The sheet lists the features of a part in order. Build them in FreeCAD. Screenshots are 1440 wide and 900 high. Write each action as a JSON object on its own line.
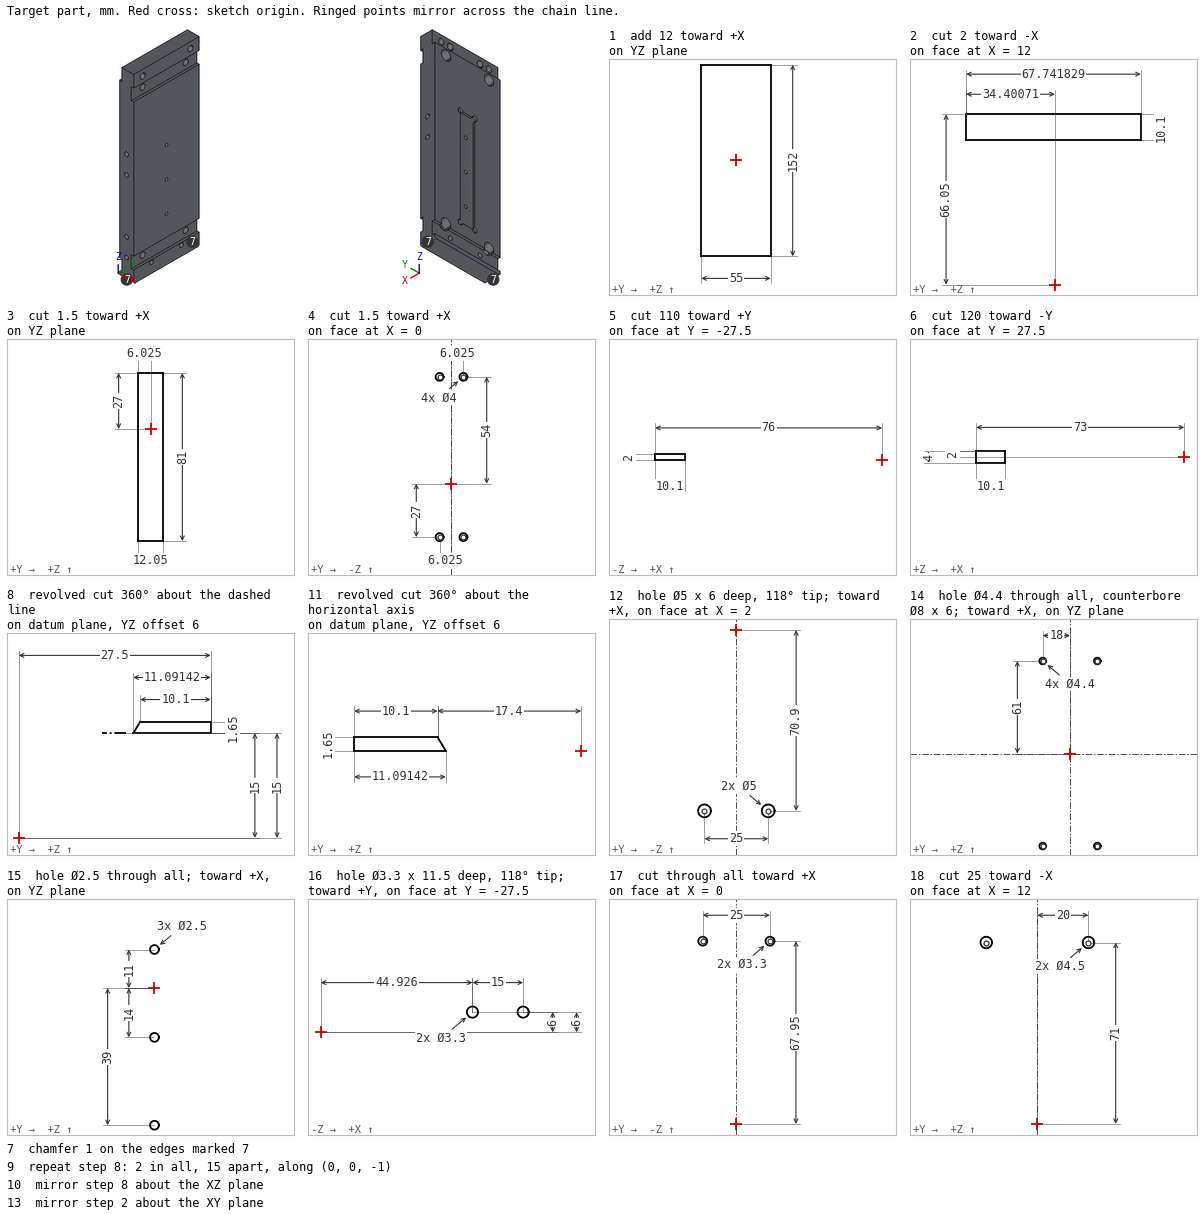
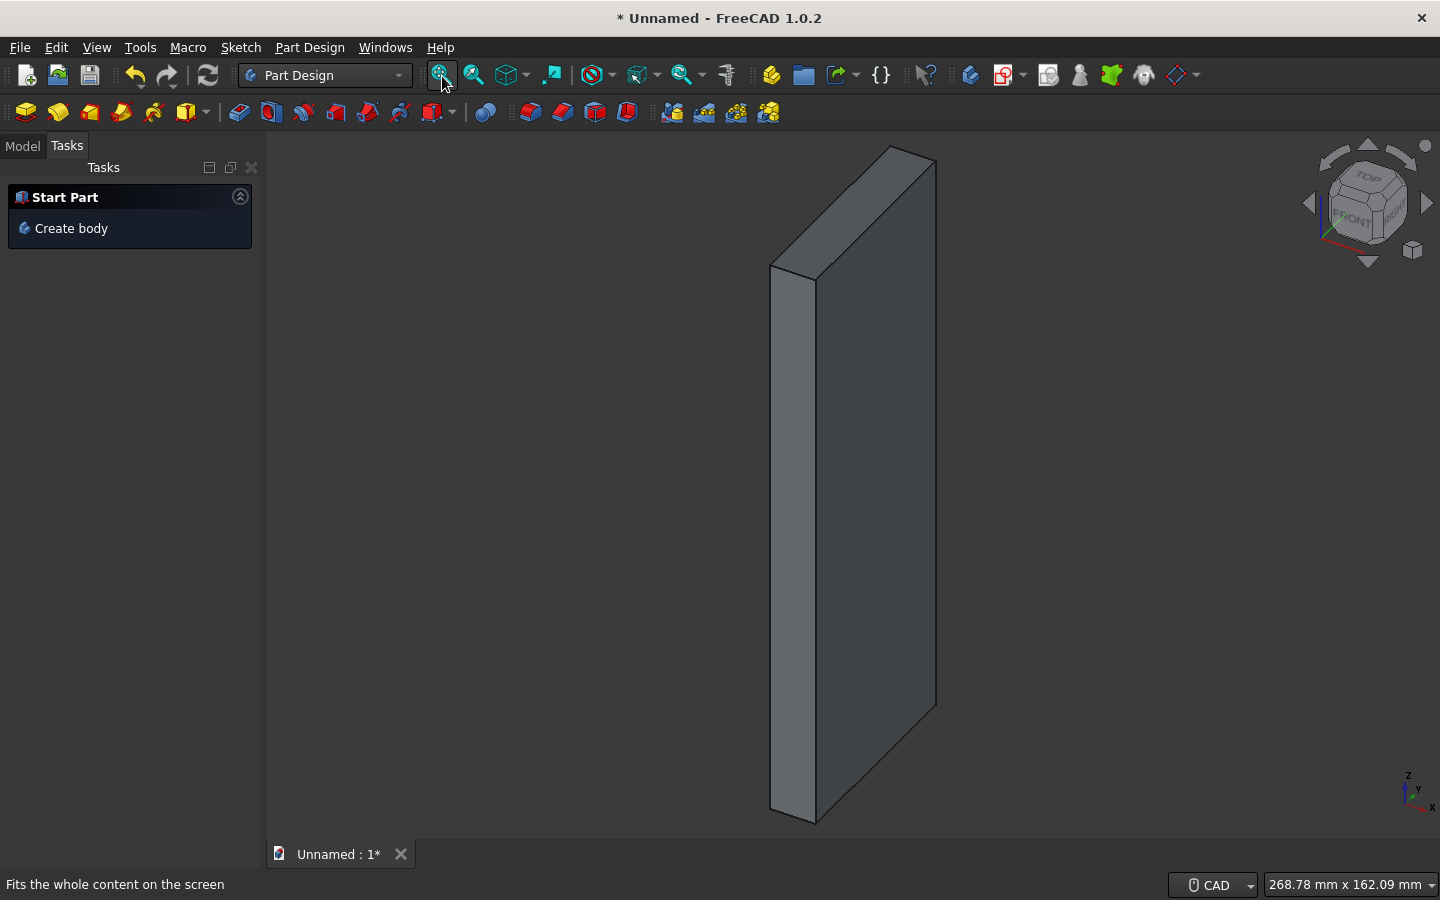
{"action": "left_click", "coordinate": [876, 647]}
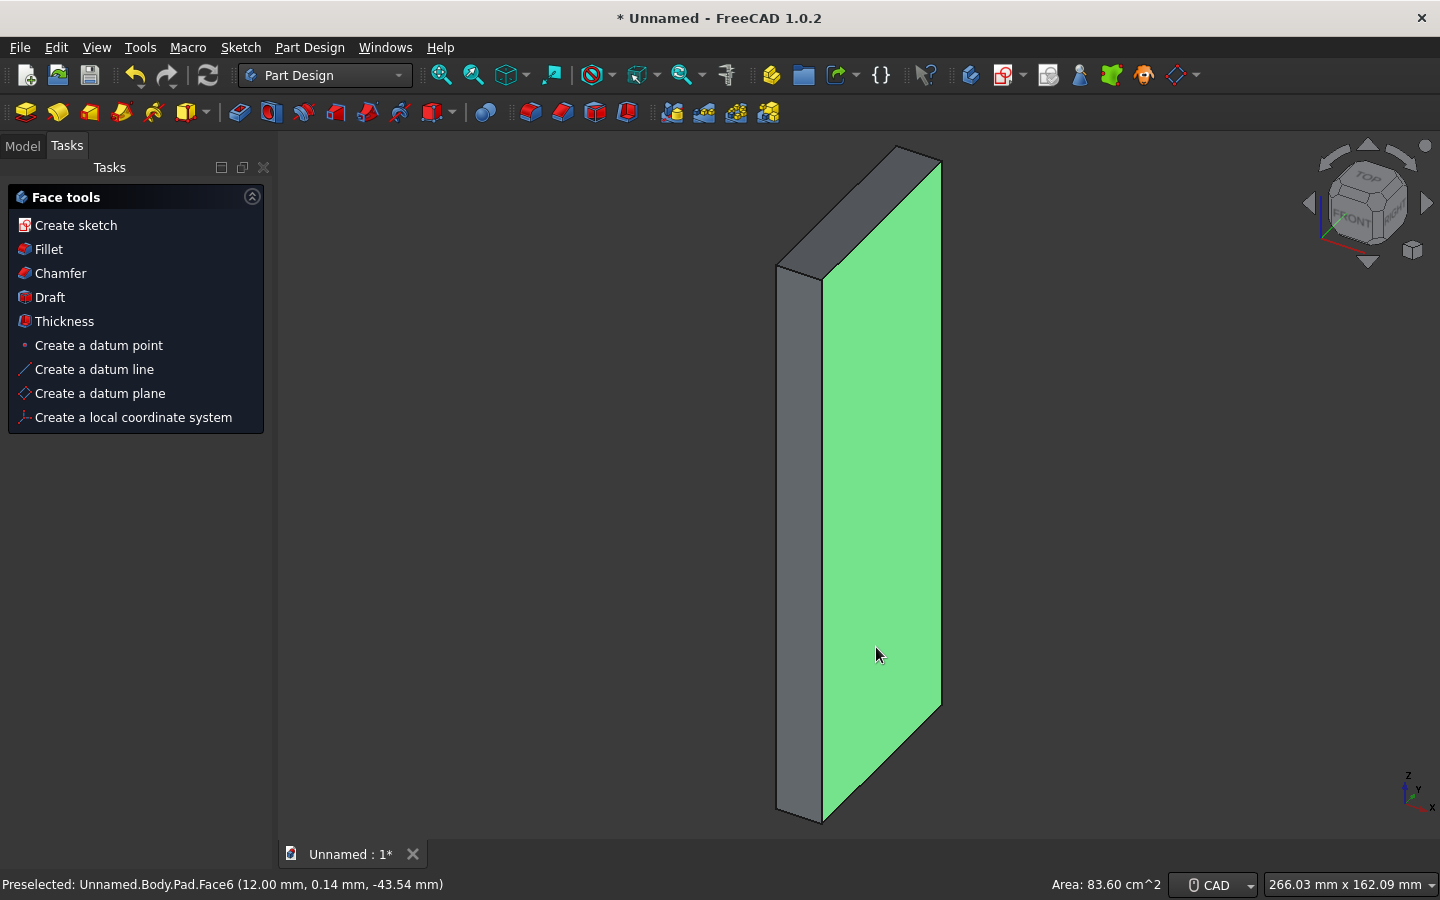
{"action": "left_click", "coordinate": [1004, 76]}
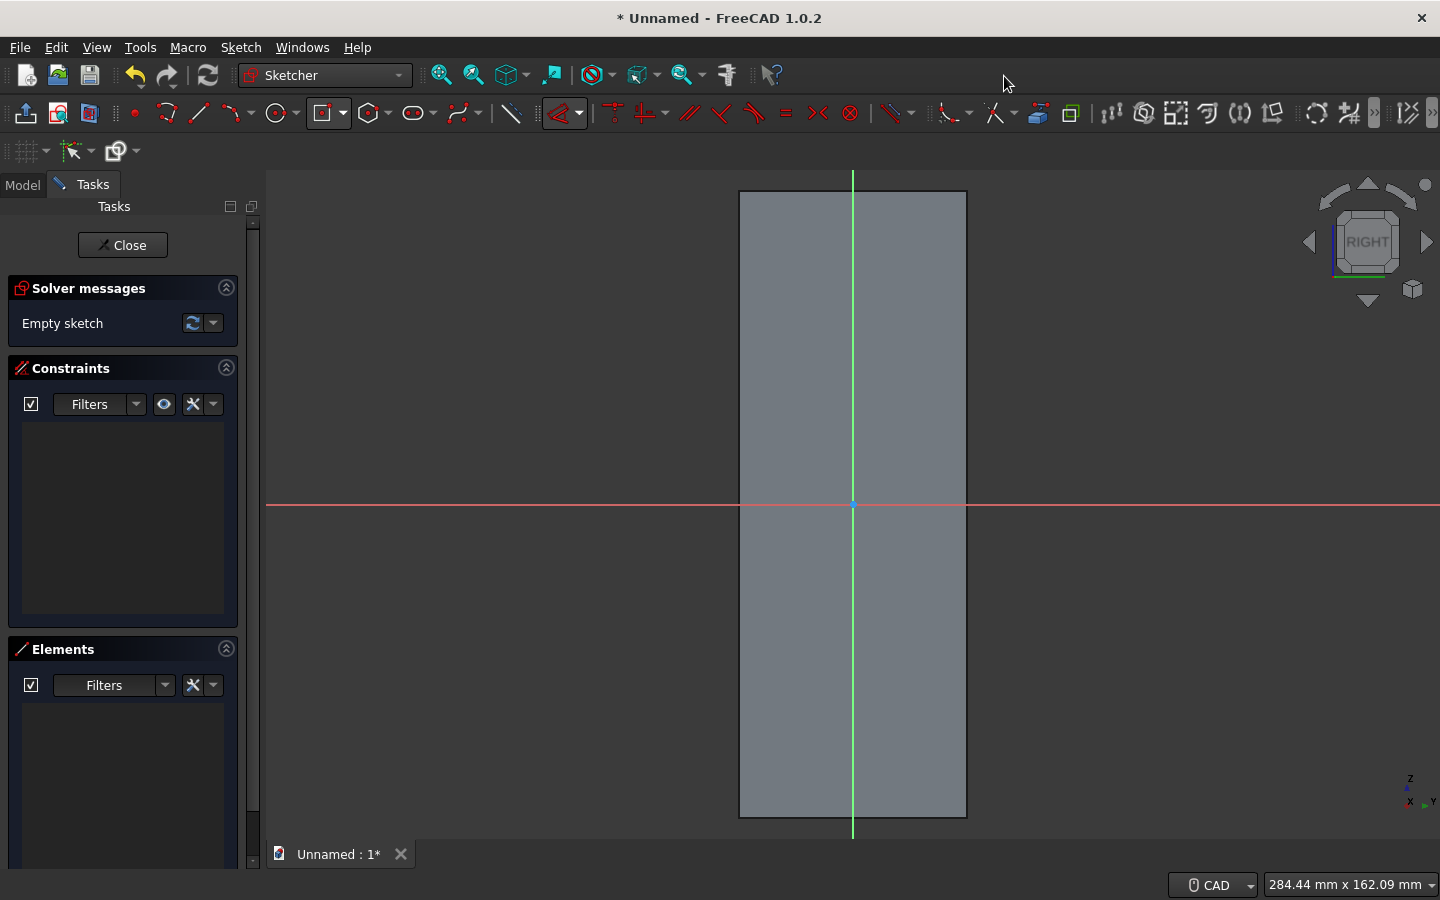
{"action": "scroll", "coordinate": [986, 198], "scroll_direction": "up", "scroll_amount": 2}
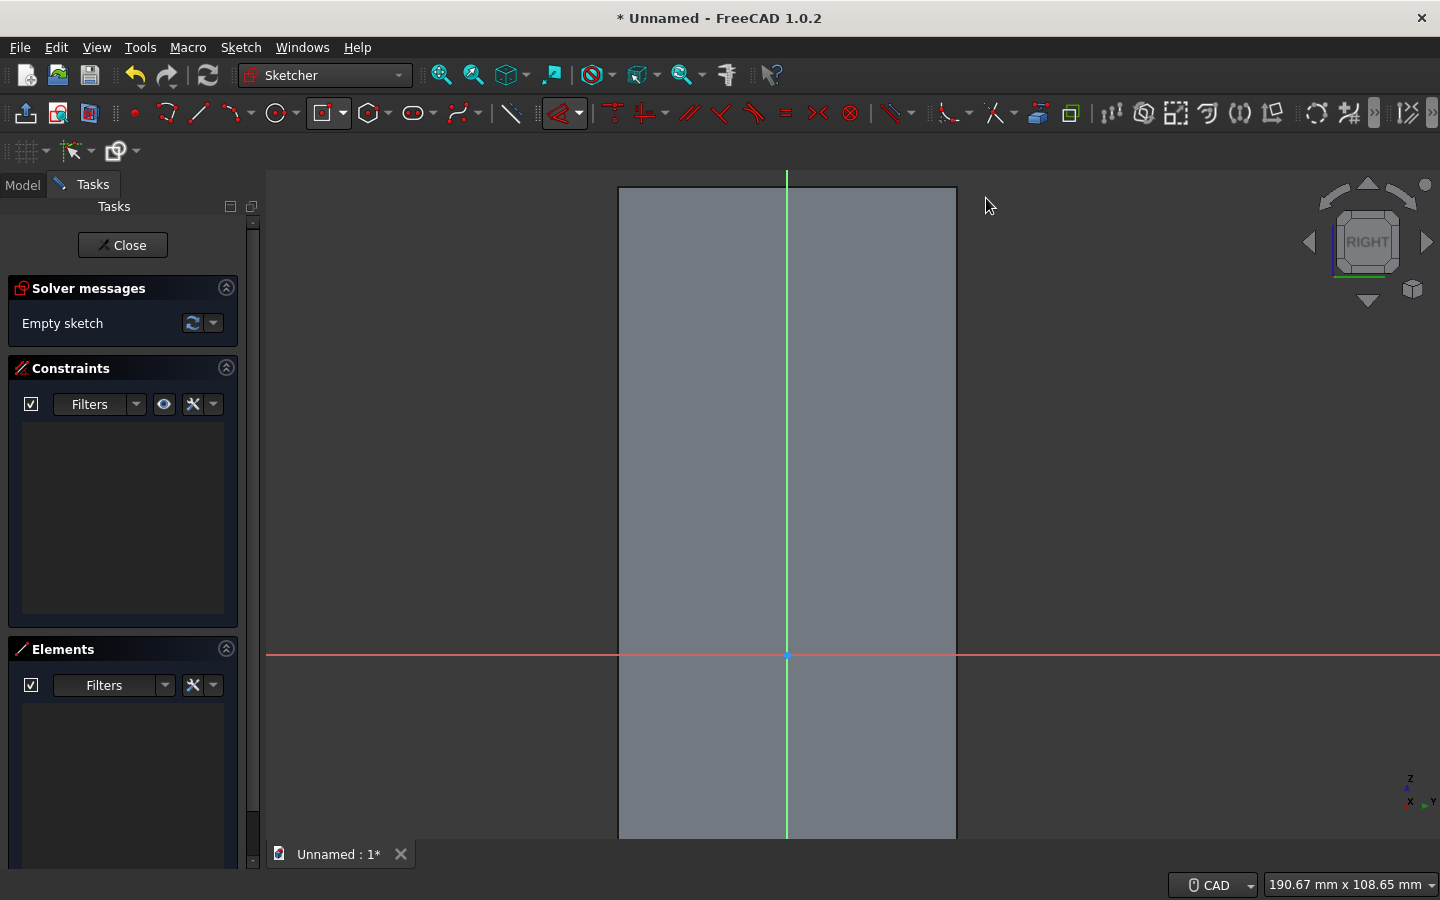
{"action": "key", "text": "g r"}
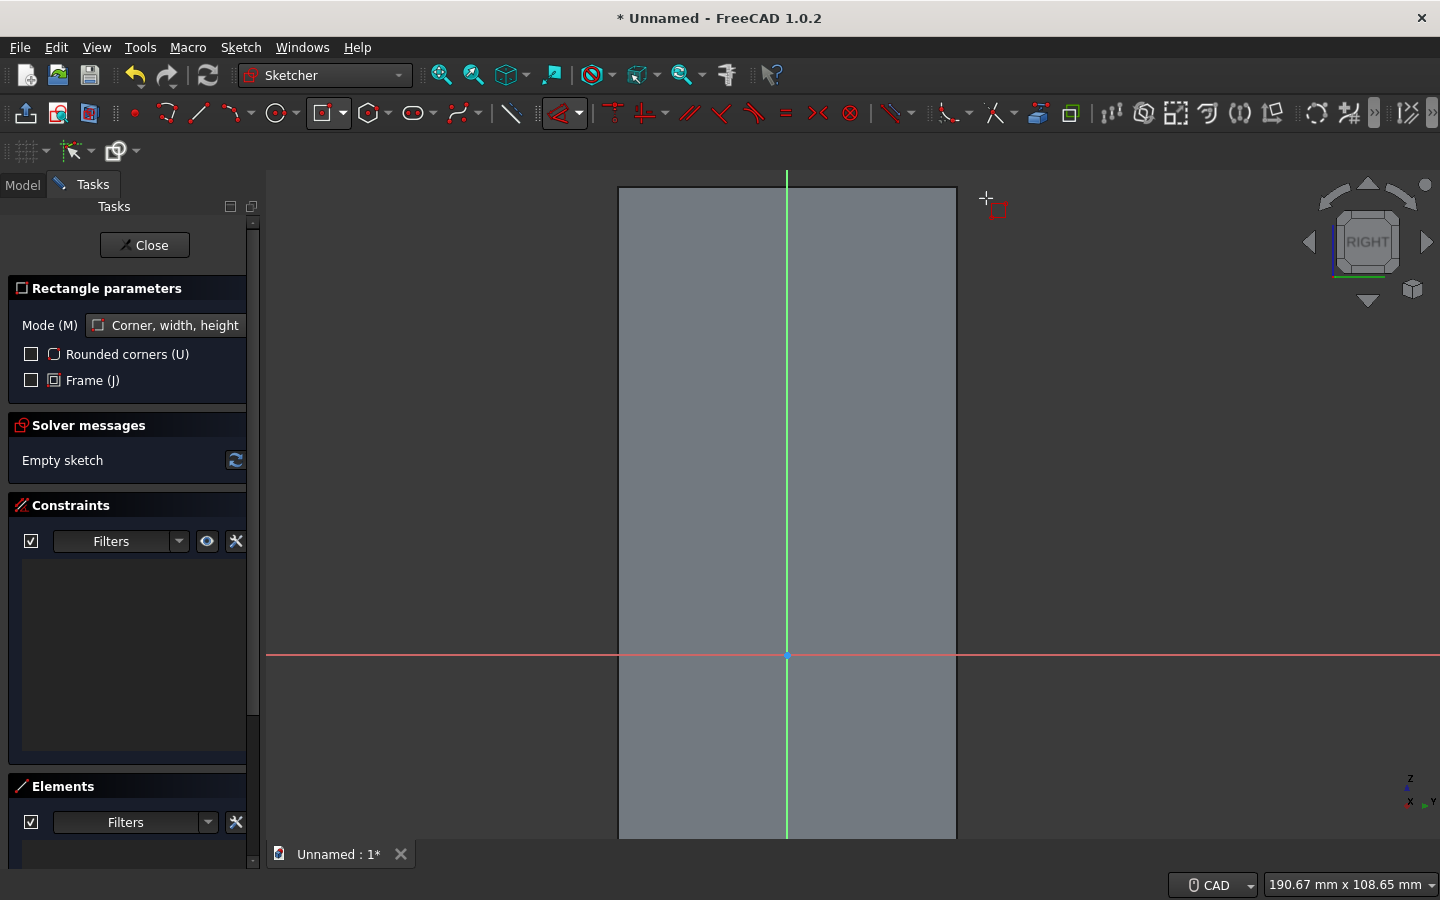
{"action": "left_click", "coordinate": [575, 249]}
{"action": "mouse_move", "coordinate": [993, 311]}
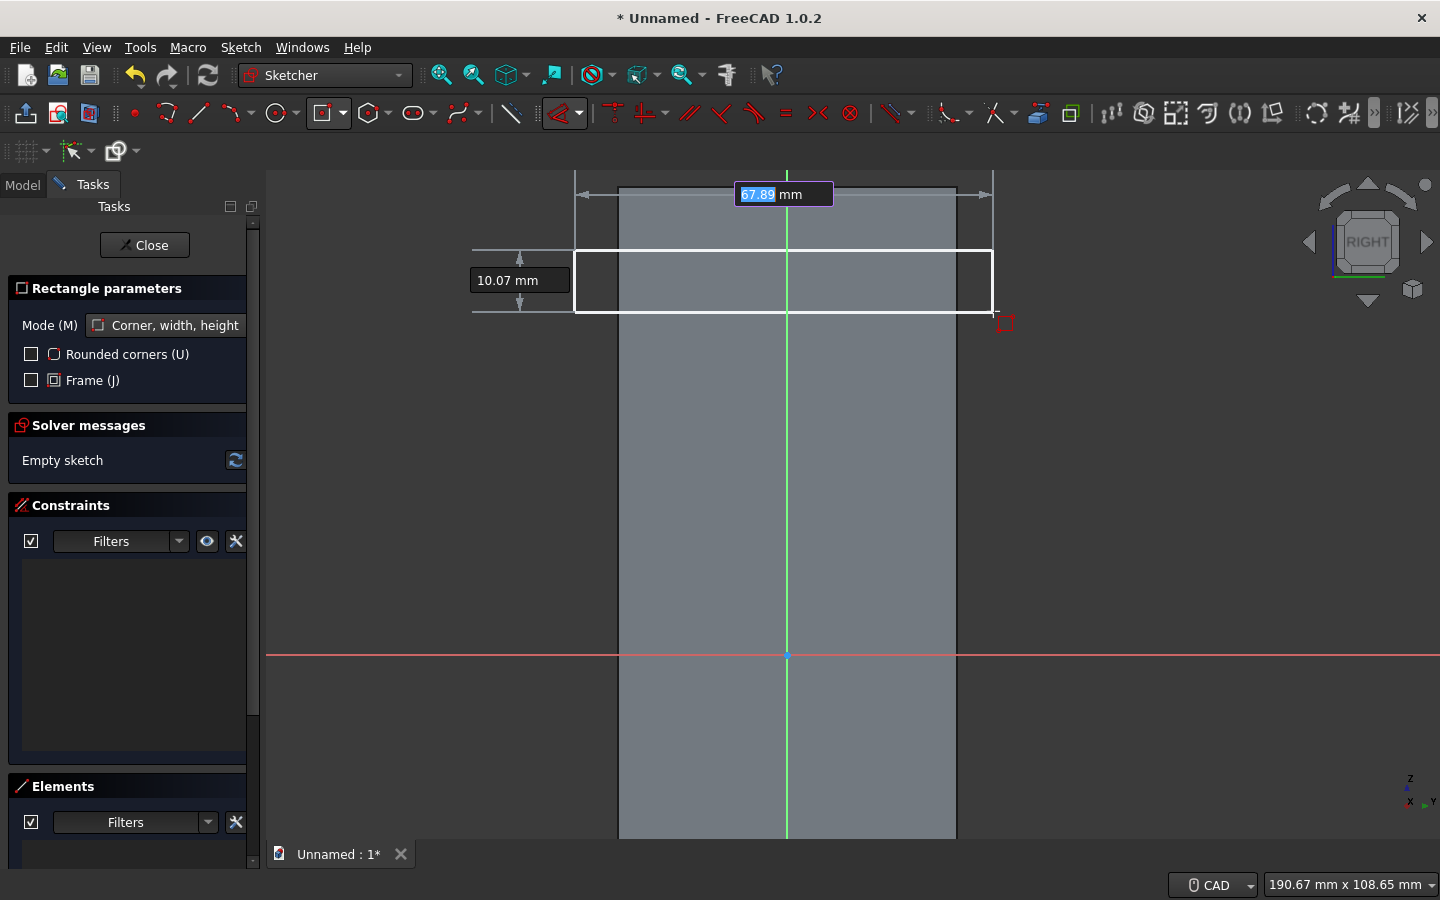
{"action": "type", "text": "67.741829"}
{"action": "key", "text": "Tab"}
{"action": "type", "text": "10.1"}
{"action": "key", "text": "Return"}
{"action": "key", "text": "Escape"}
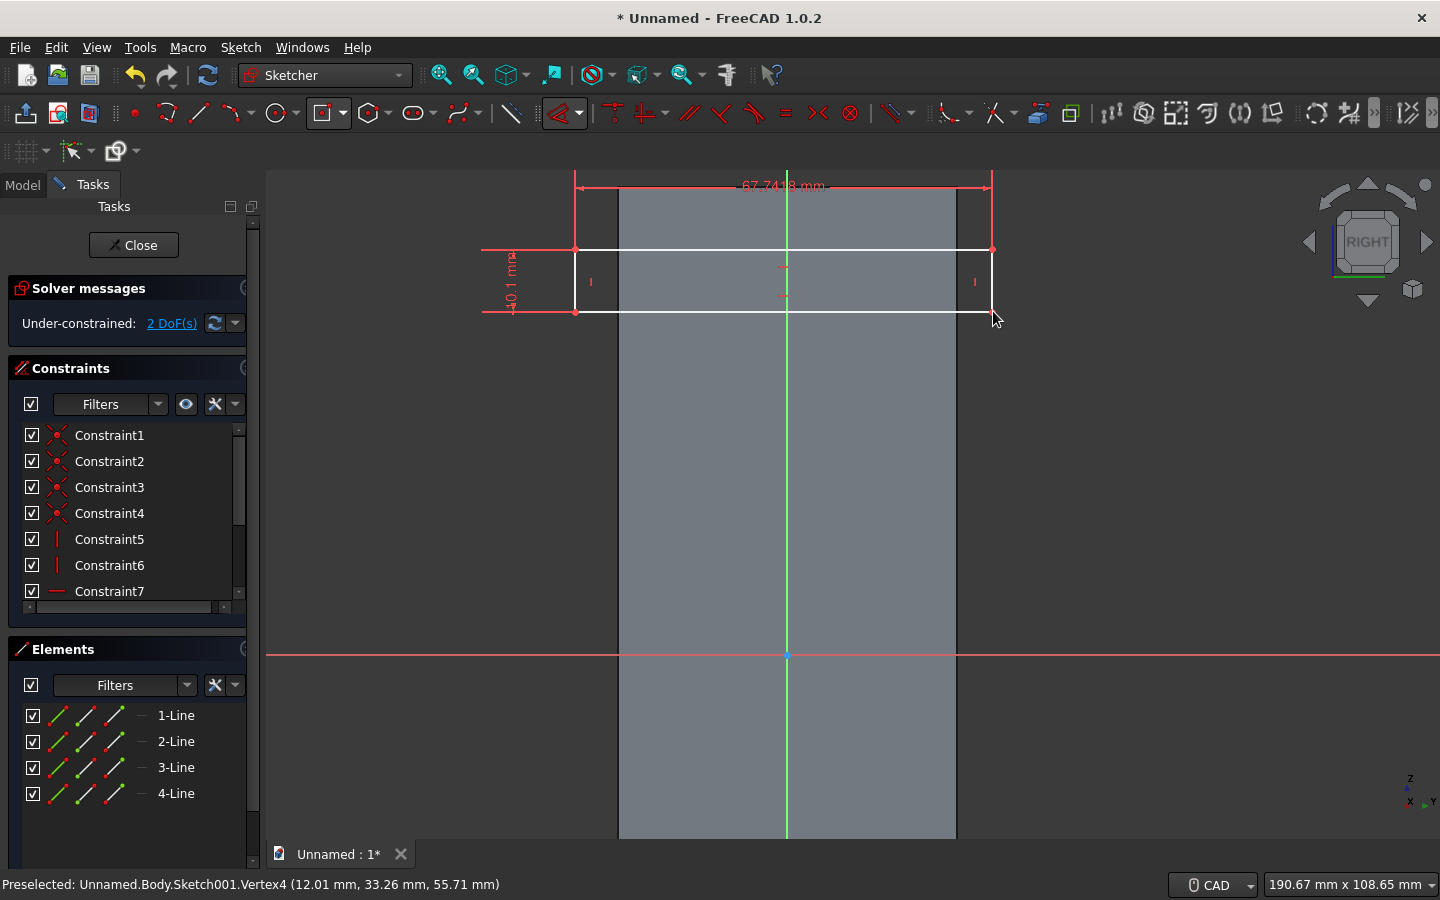
{"action": "left_click", "coordinate": [575, 250]}